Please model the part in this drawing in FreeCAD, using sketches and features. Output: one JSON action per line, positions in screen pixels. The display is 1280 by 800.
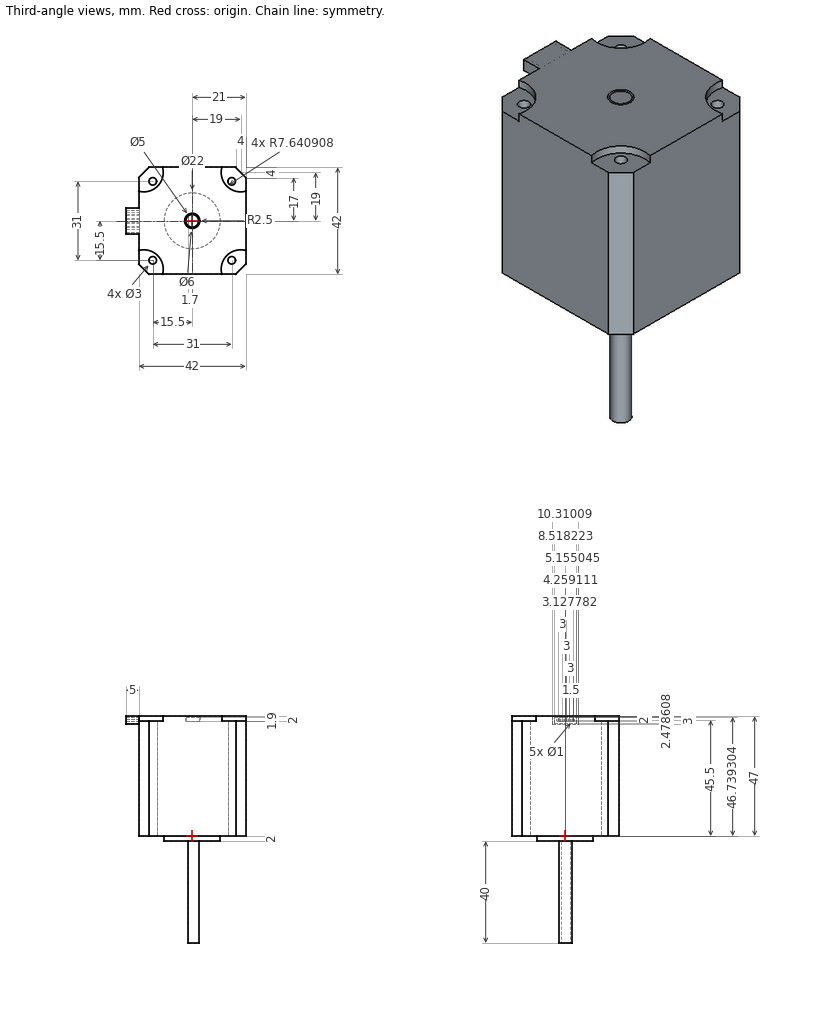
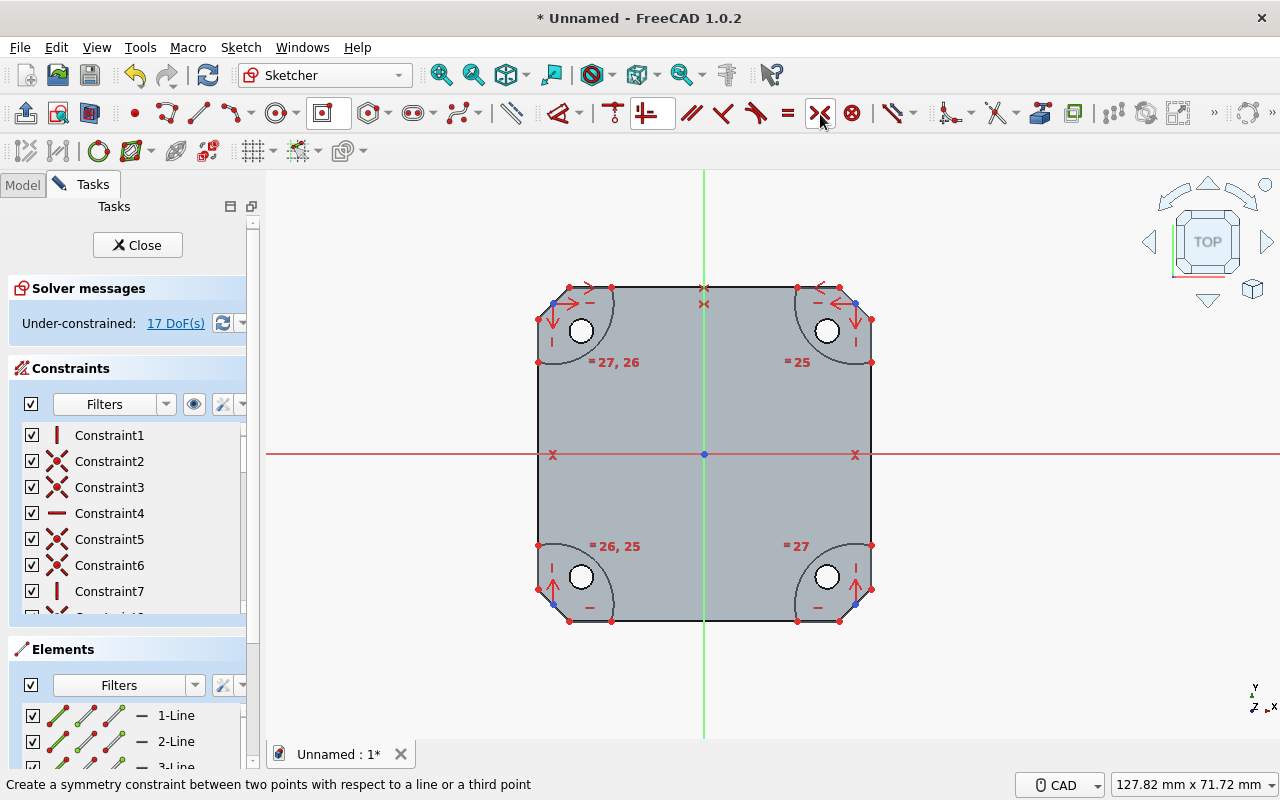
{"action": "left_click", "coordinate": [569, 622]}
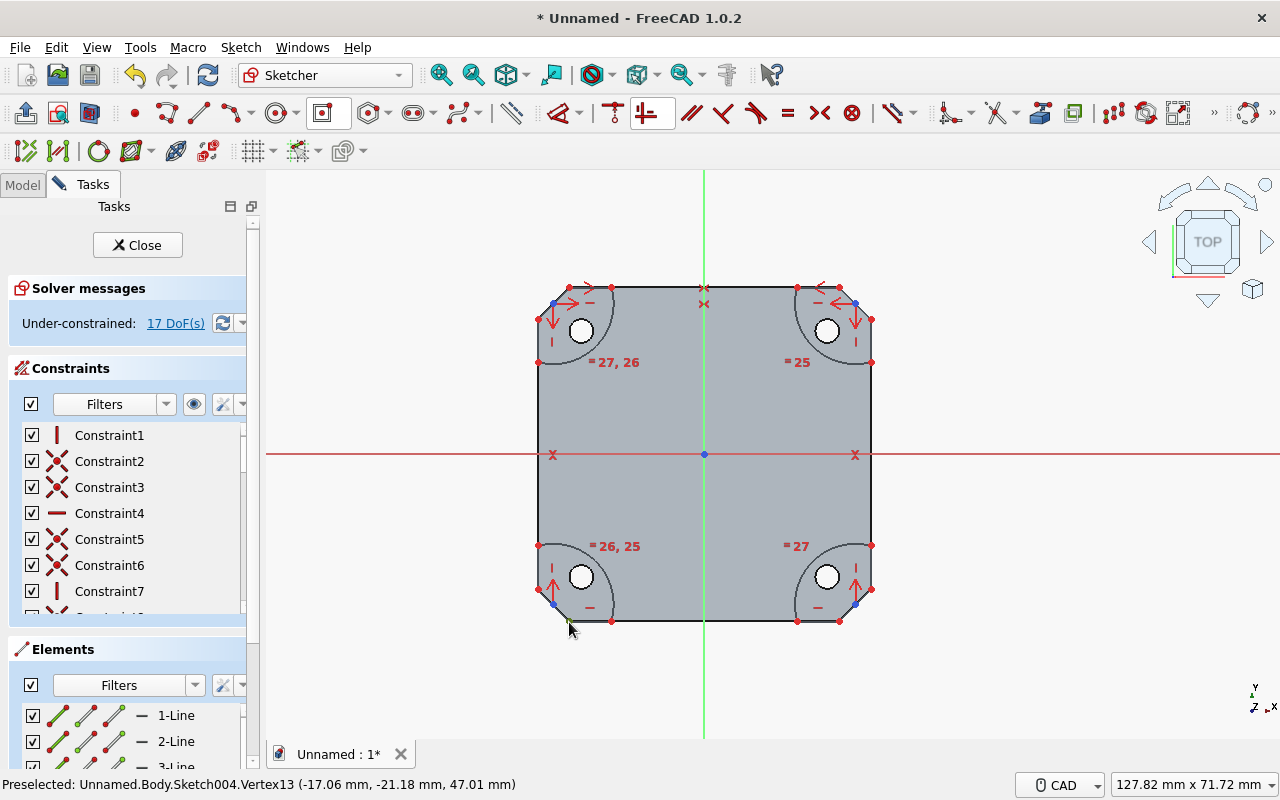
{"action": "left_click", "coordinate": [570, 288]}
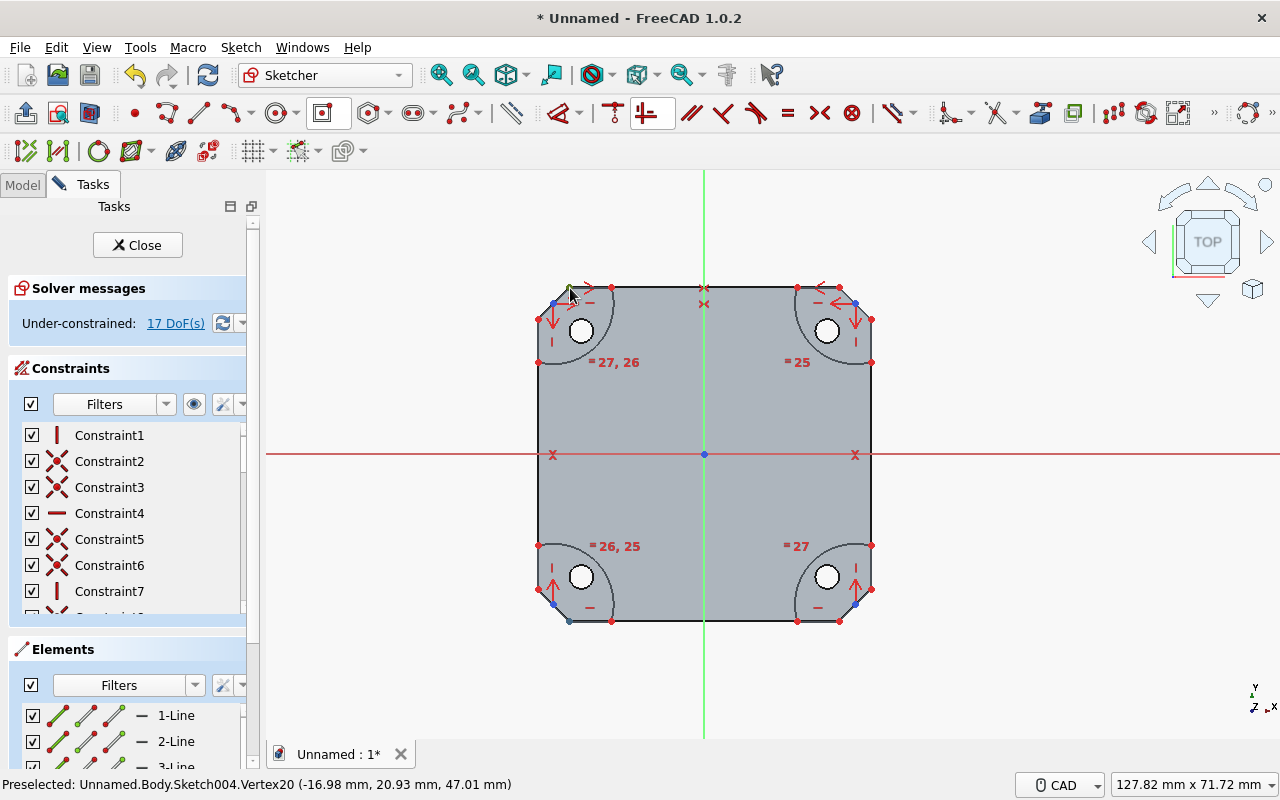
{"action": "left_click", "coordinate": [353, 454]}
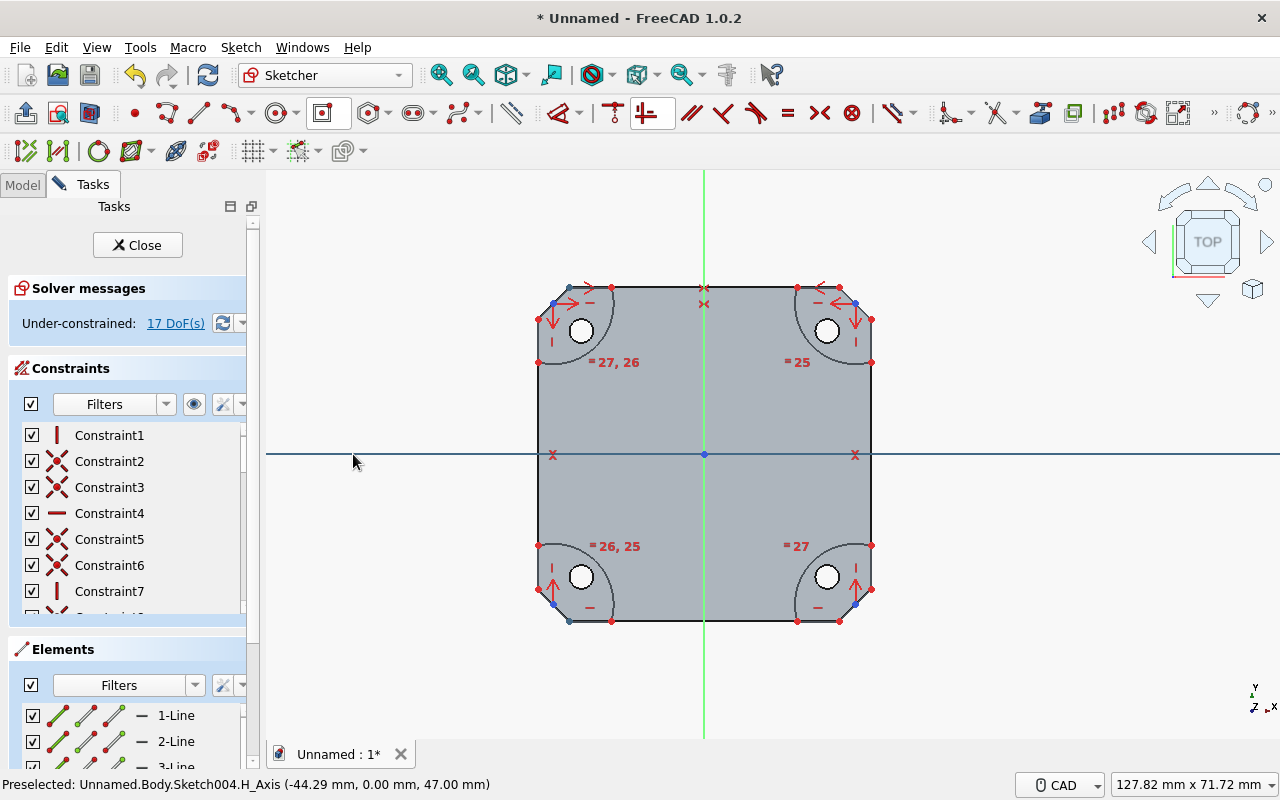
{"action": "key", "text": "s"}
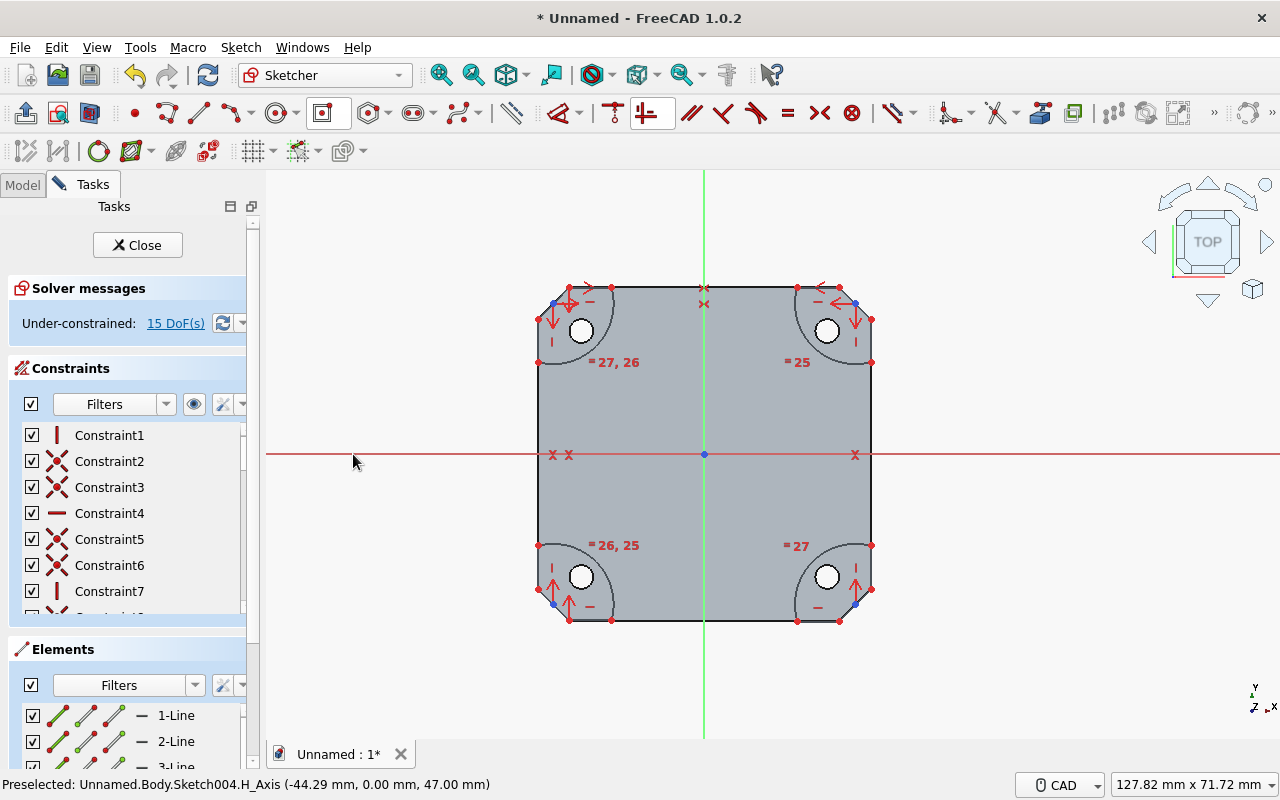
{"action": "left_click", "coordinate": [871, 320]}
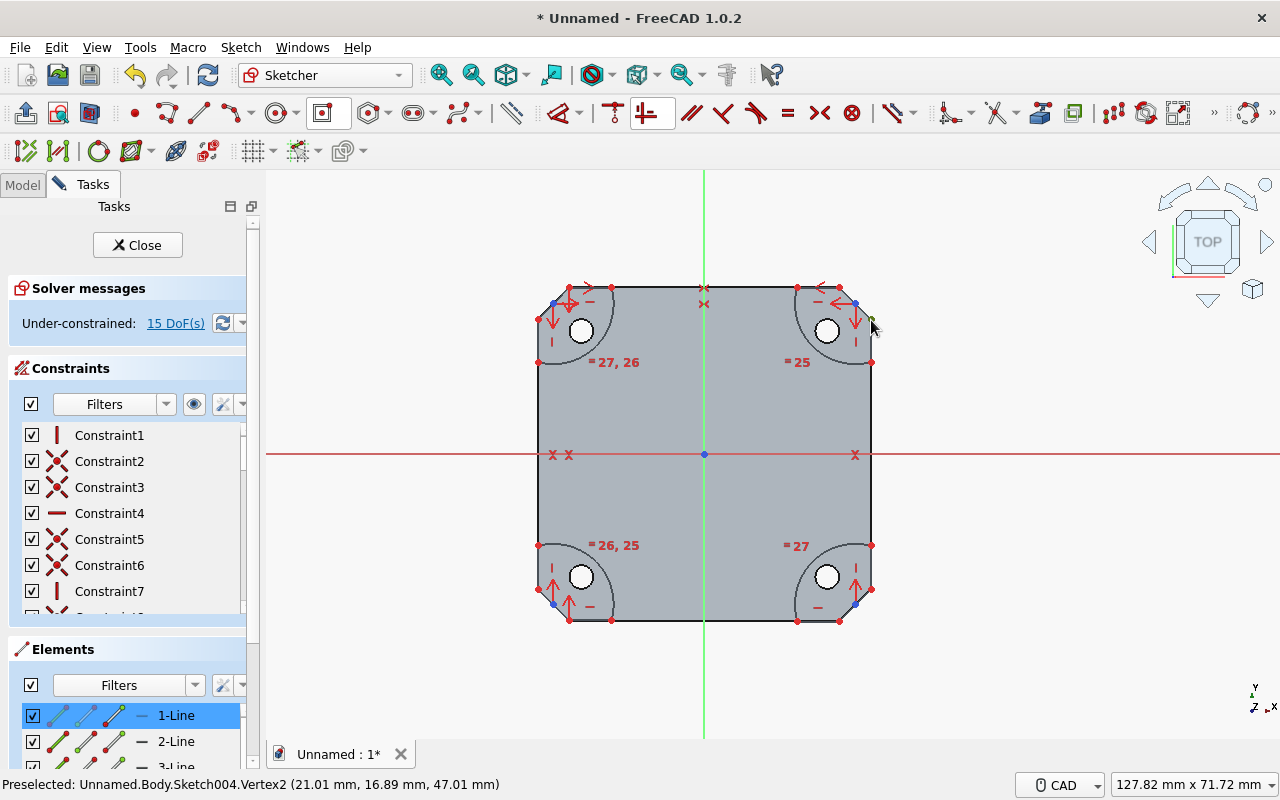
{"action": "left_click", "coordinate": [538, 320]}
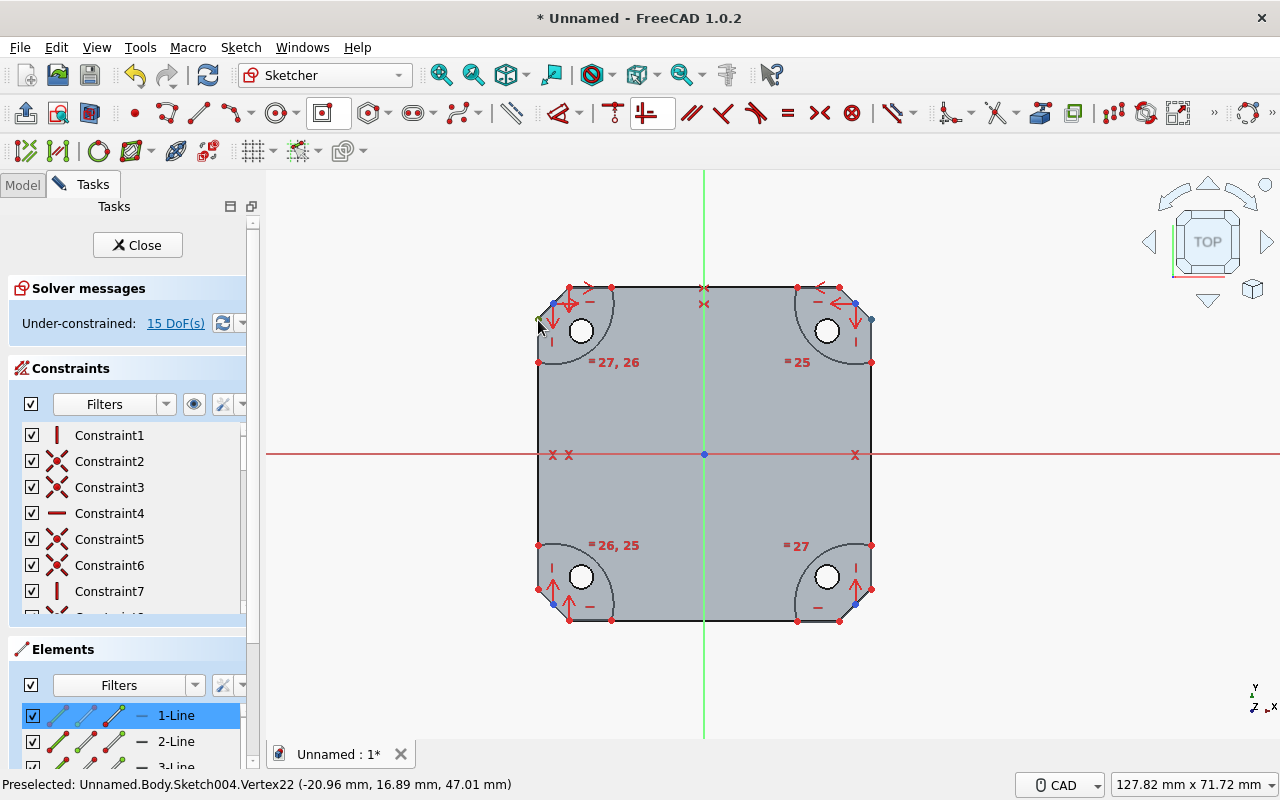
{"action": "left_click", "coordinate": [704, 674]}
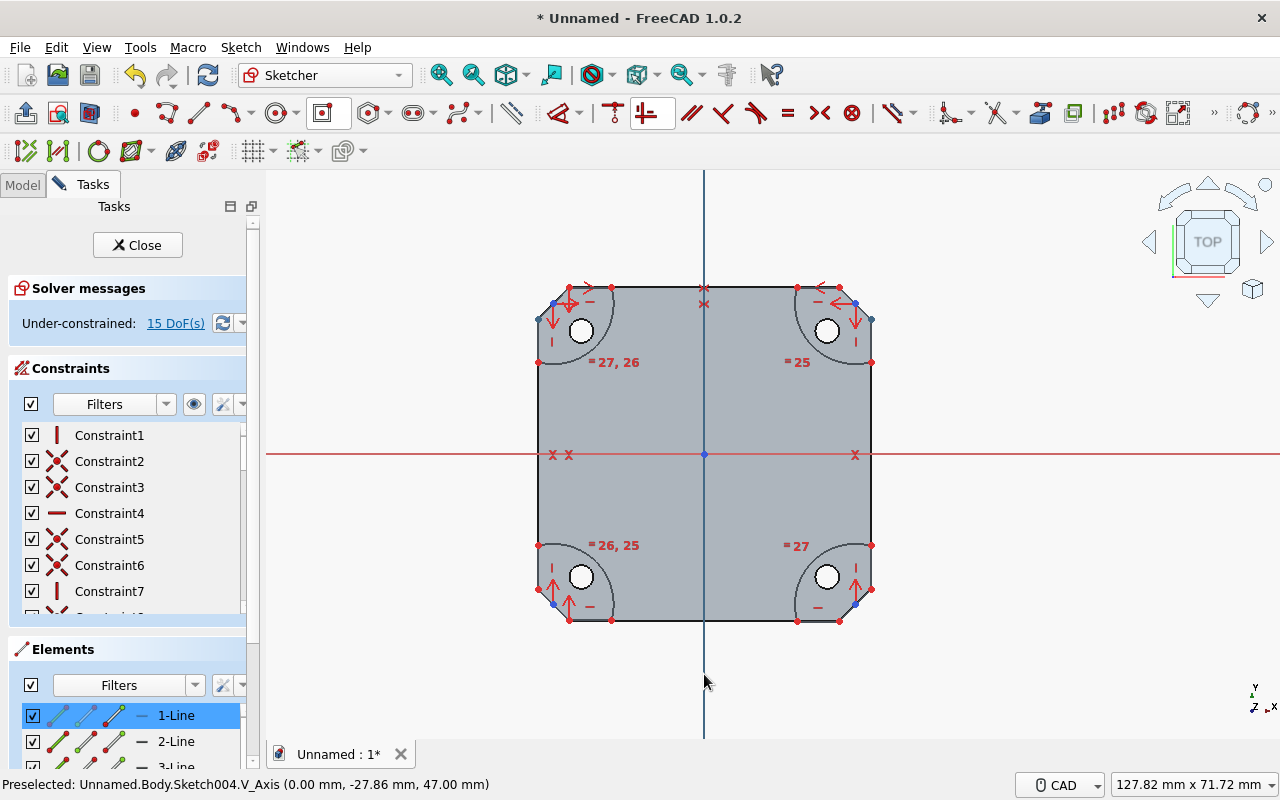
{"action": "left_click", "coordinate": [820, 114]}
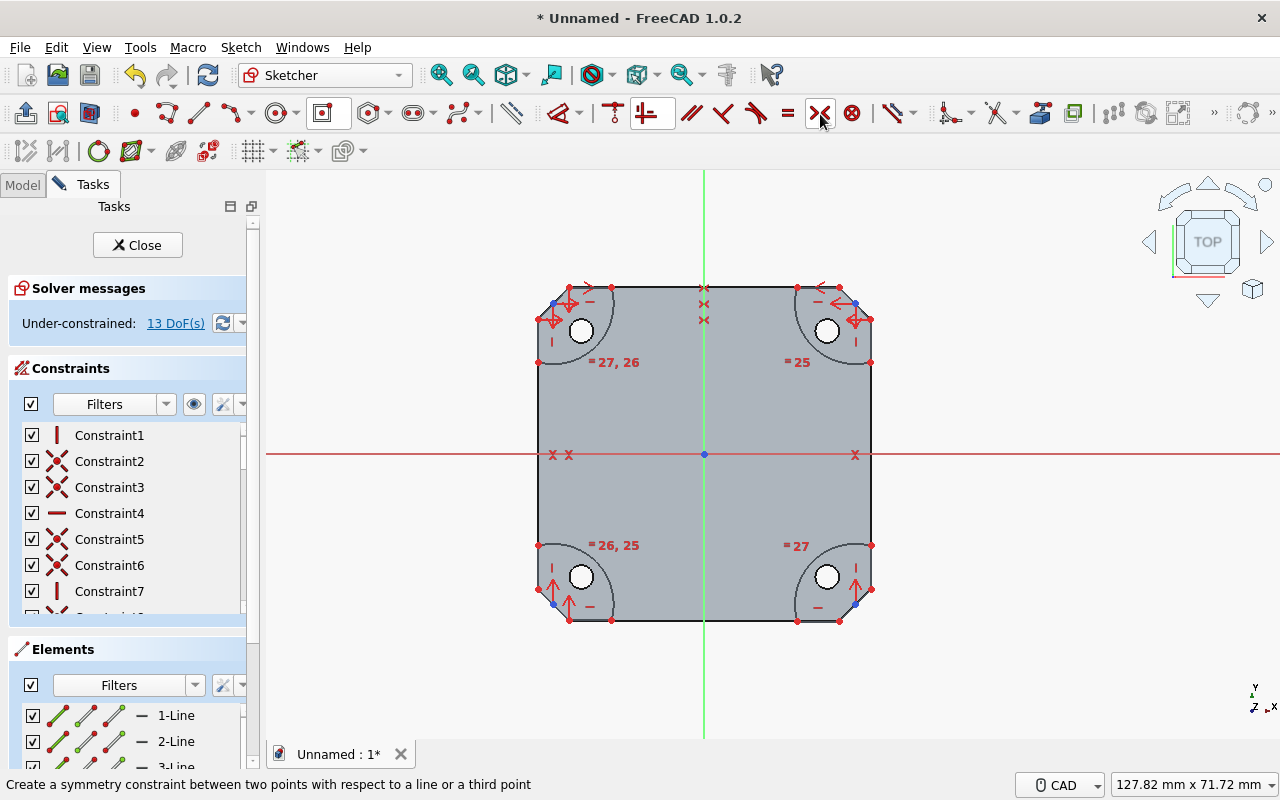
{"action": "left_click", "coordinate": [538, 590]}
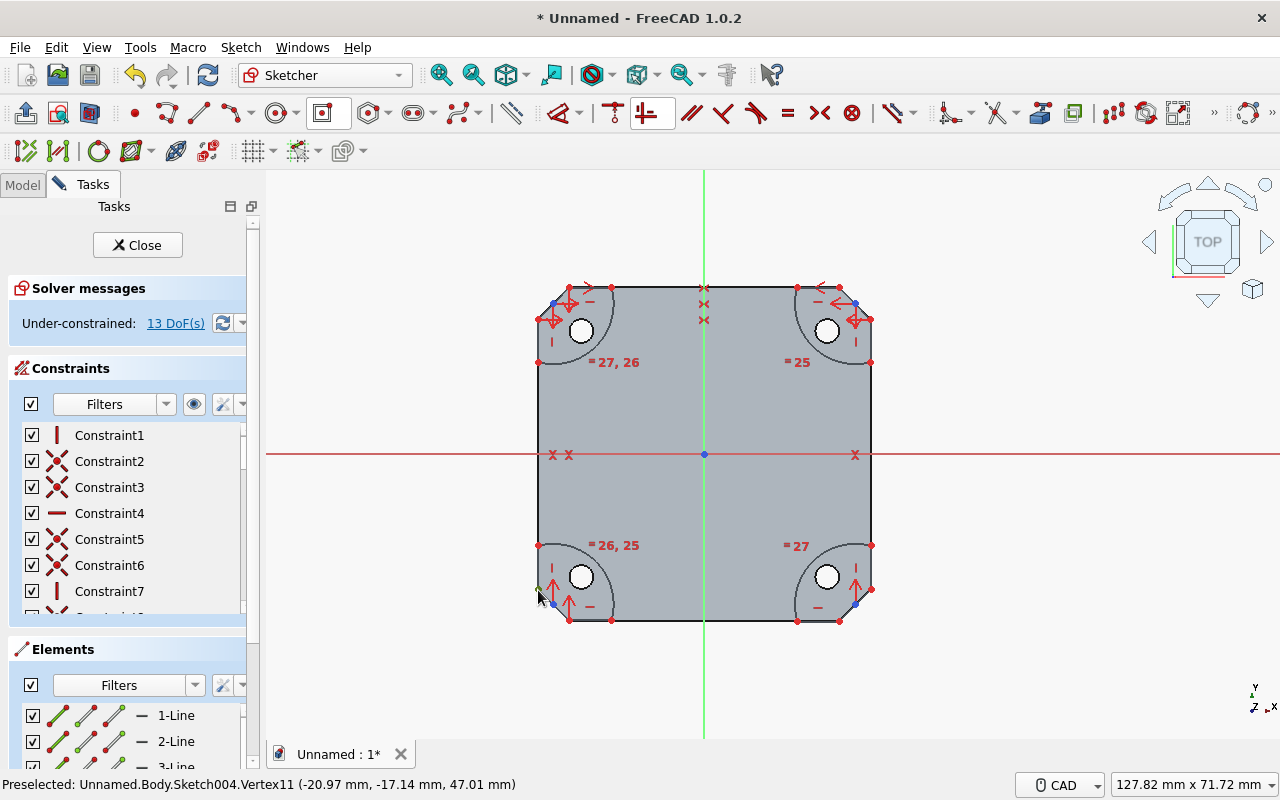
{"action": "left_click", "coordinate": [538, 320]}